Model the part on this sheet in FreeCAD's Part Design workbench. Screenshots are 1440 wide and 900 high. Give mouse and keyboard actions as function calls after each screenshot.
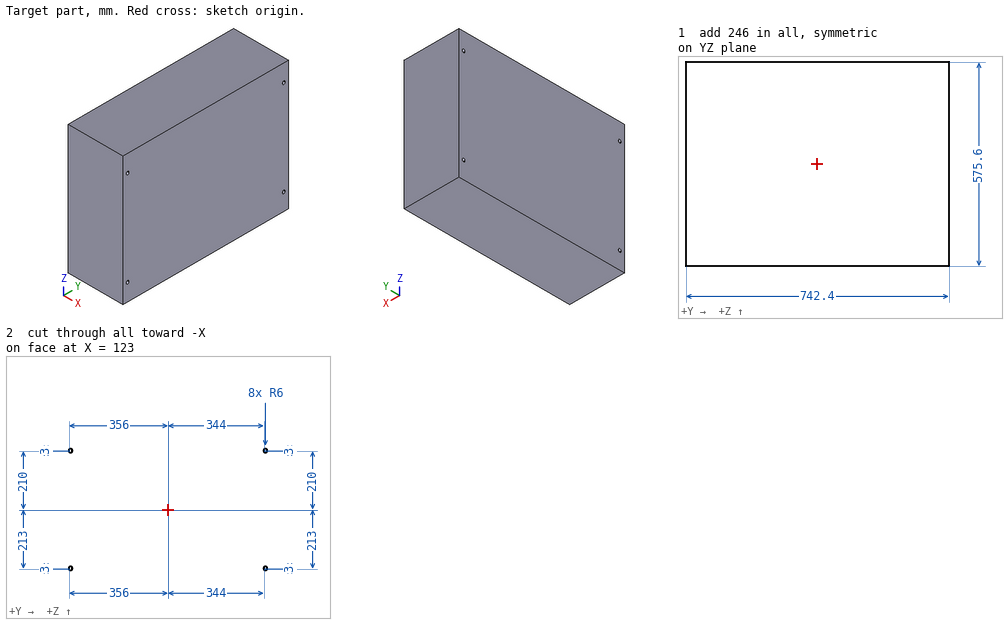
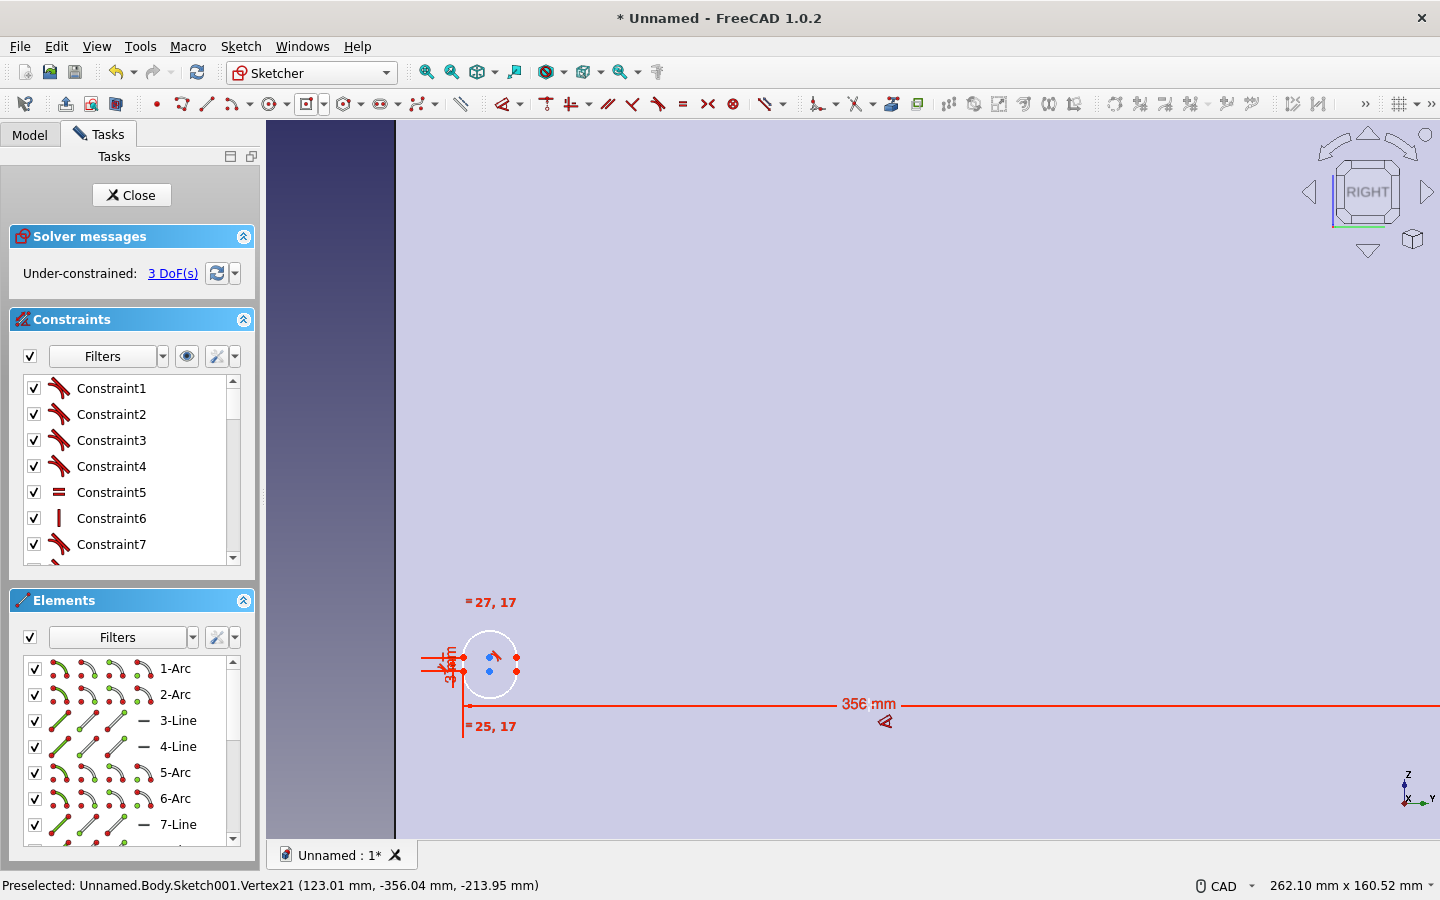
click(463, 671)
click(429, 410)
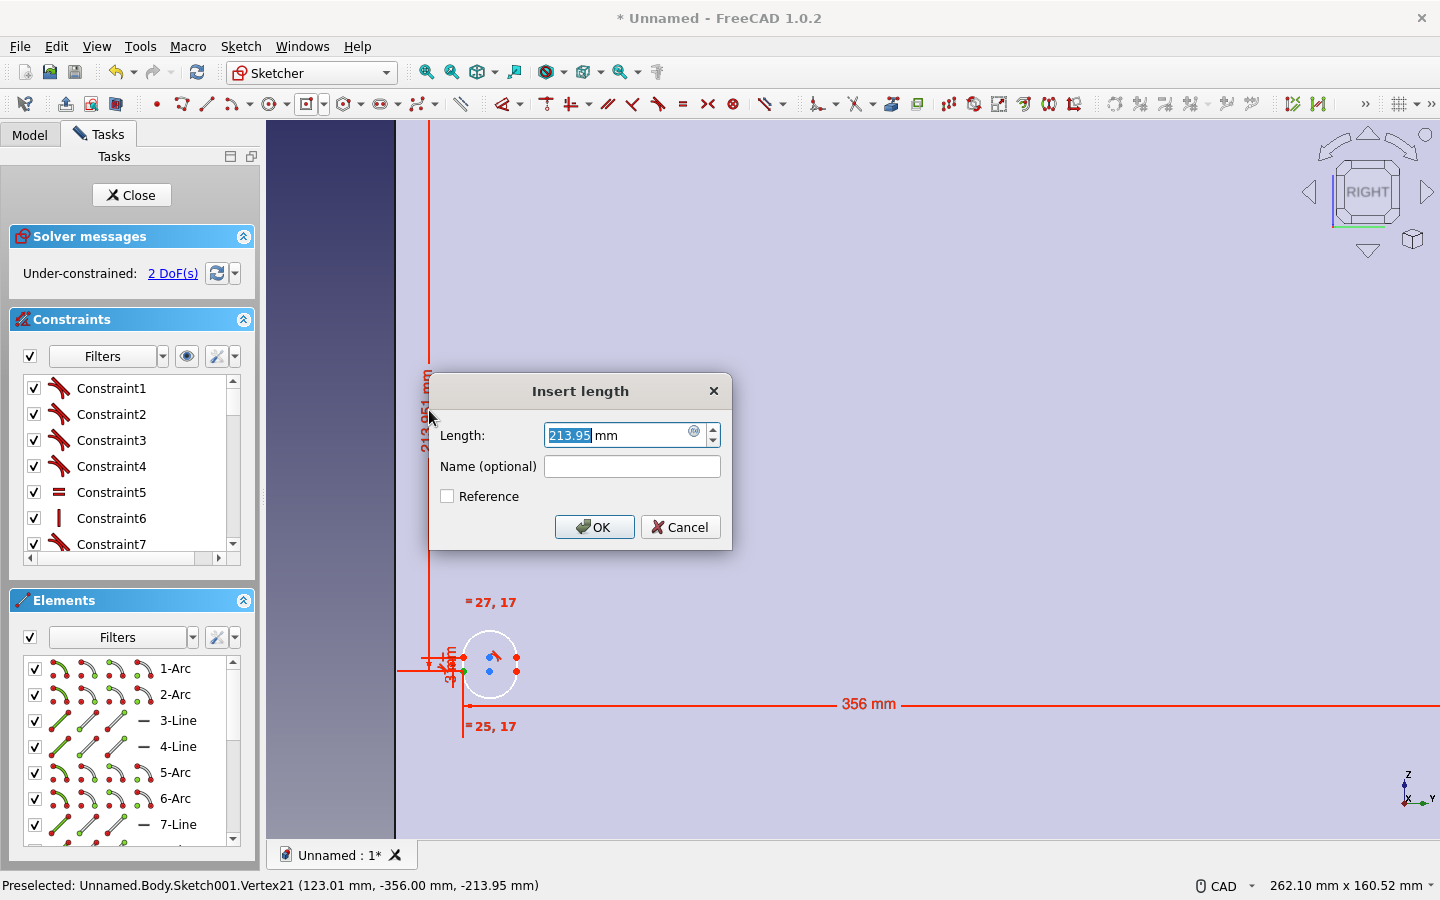
text(213)
key(Return)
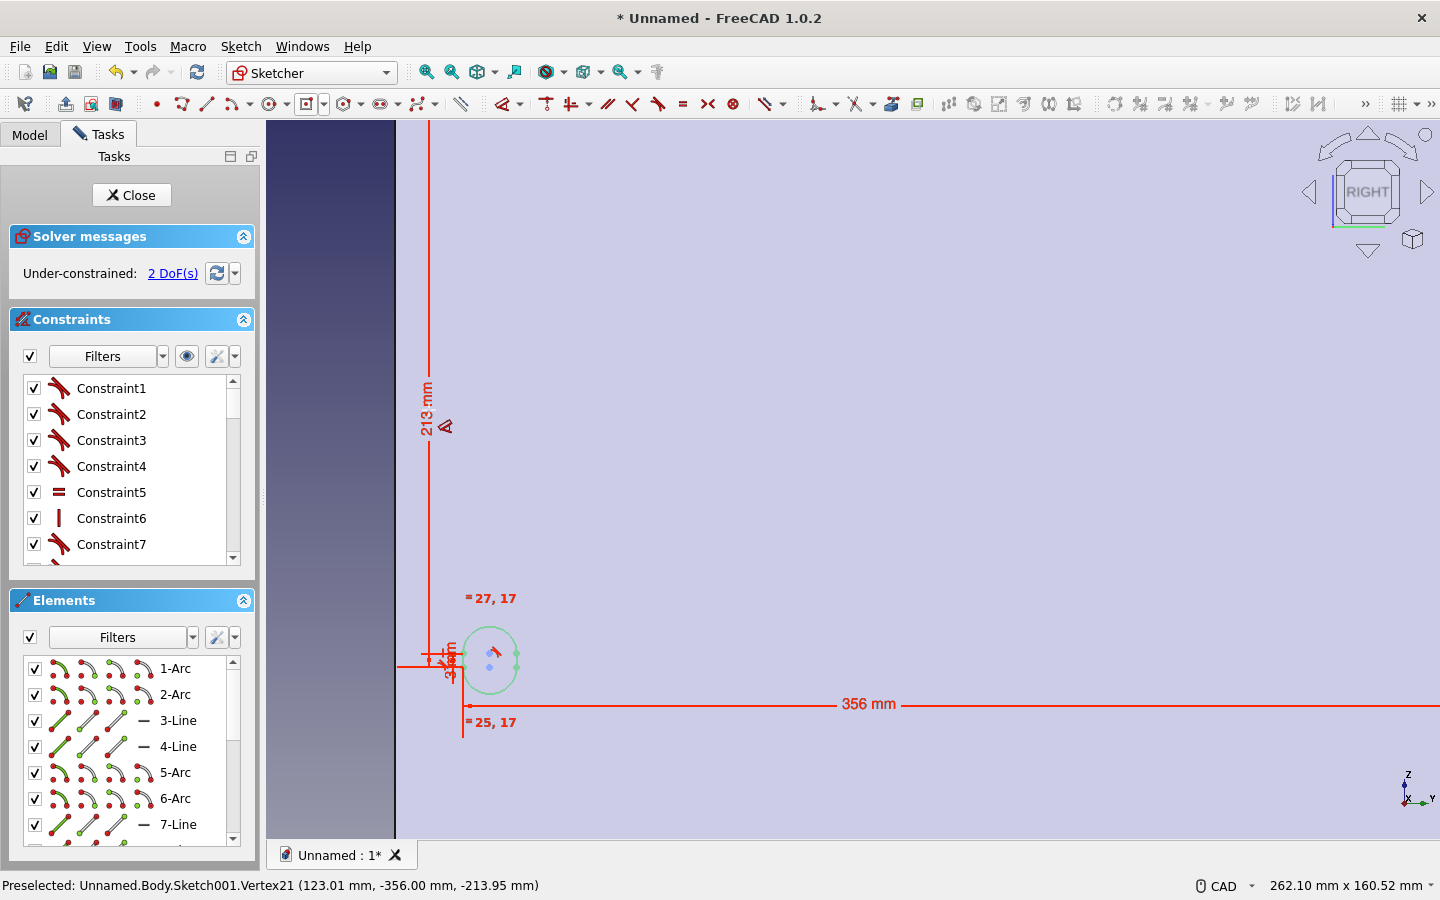
scroll(462, 673, down, 8)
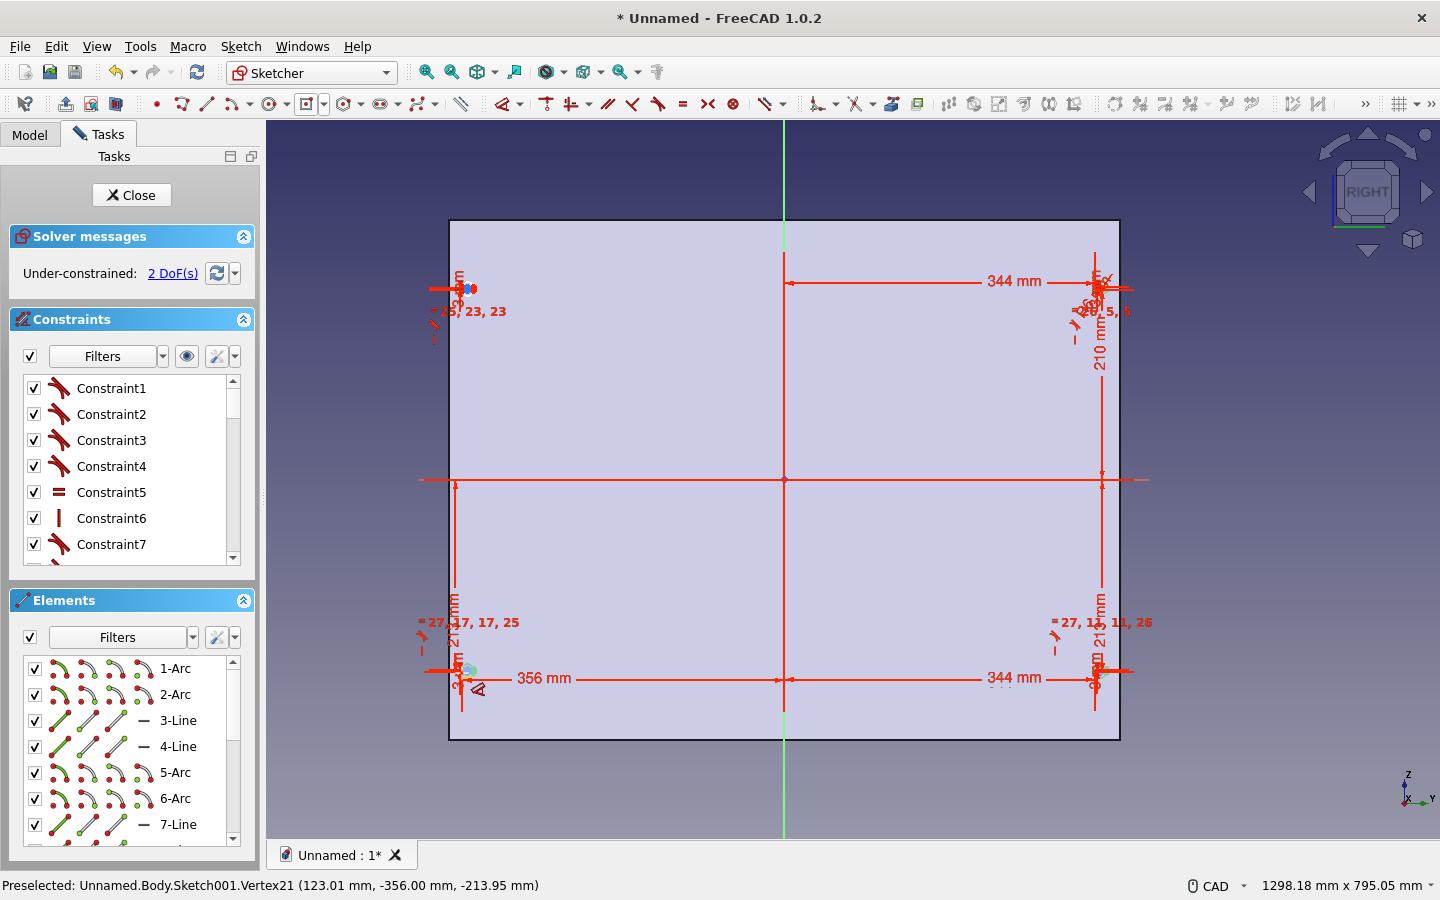
scroll(463, 290, up, 8)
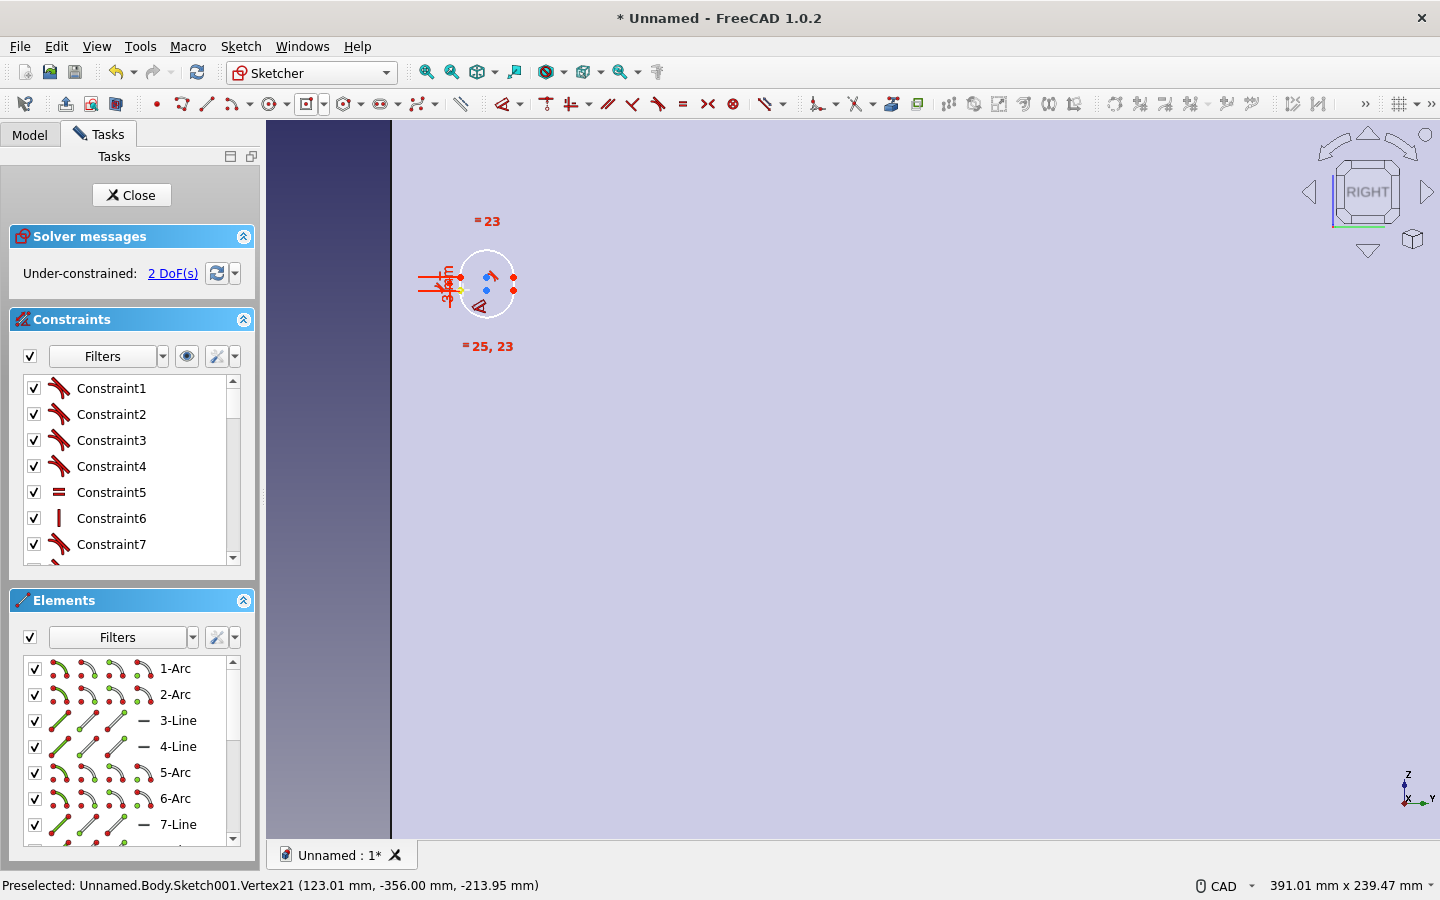
click(460, 291)
click(868, 257)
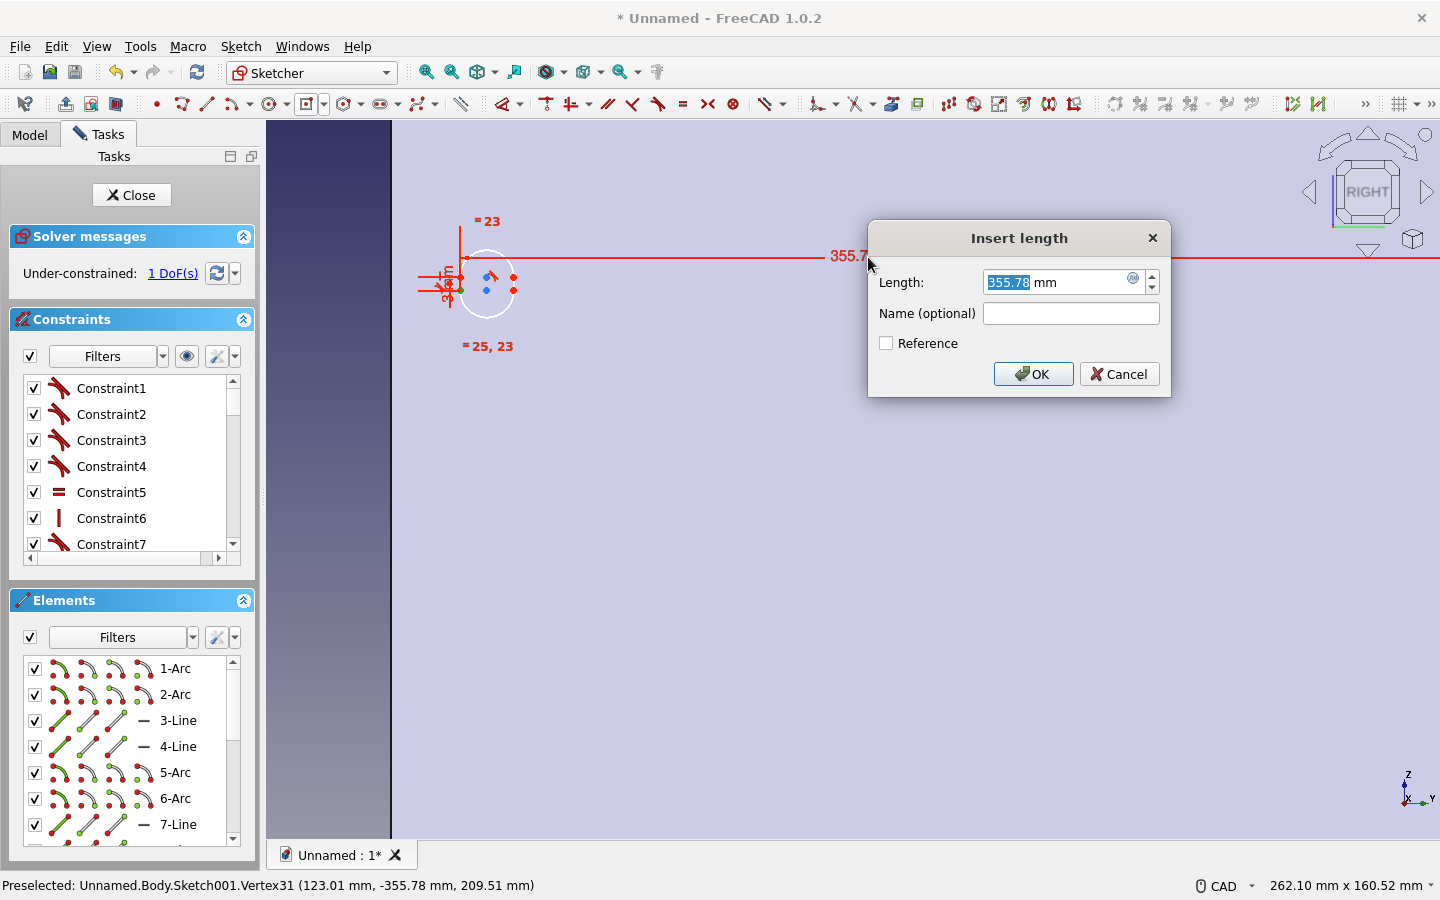
text(356)
key(Return)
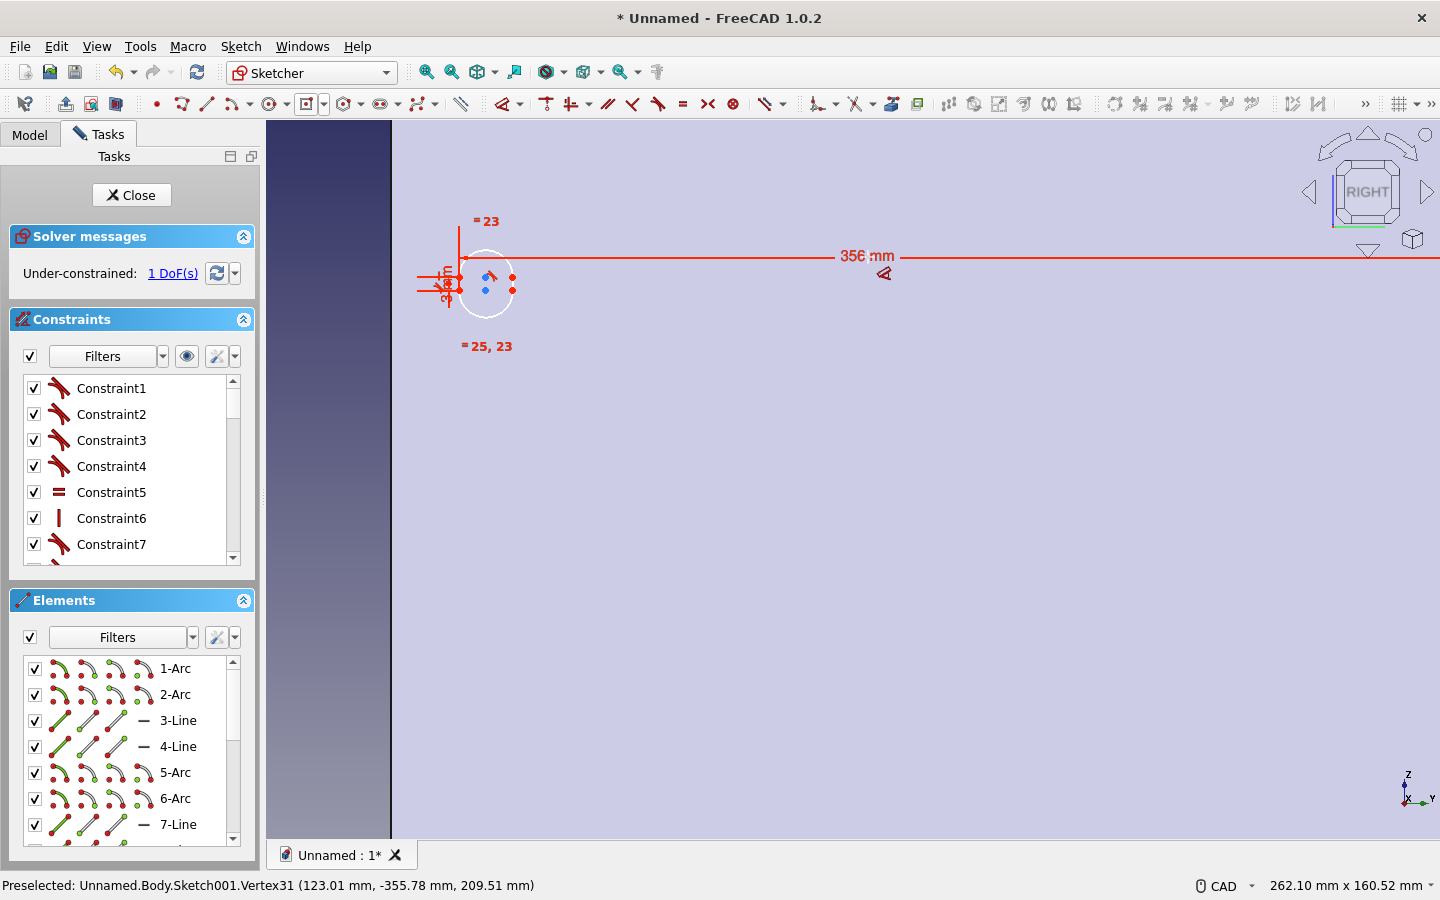
click(459, 291)
click(425, 551)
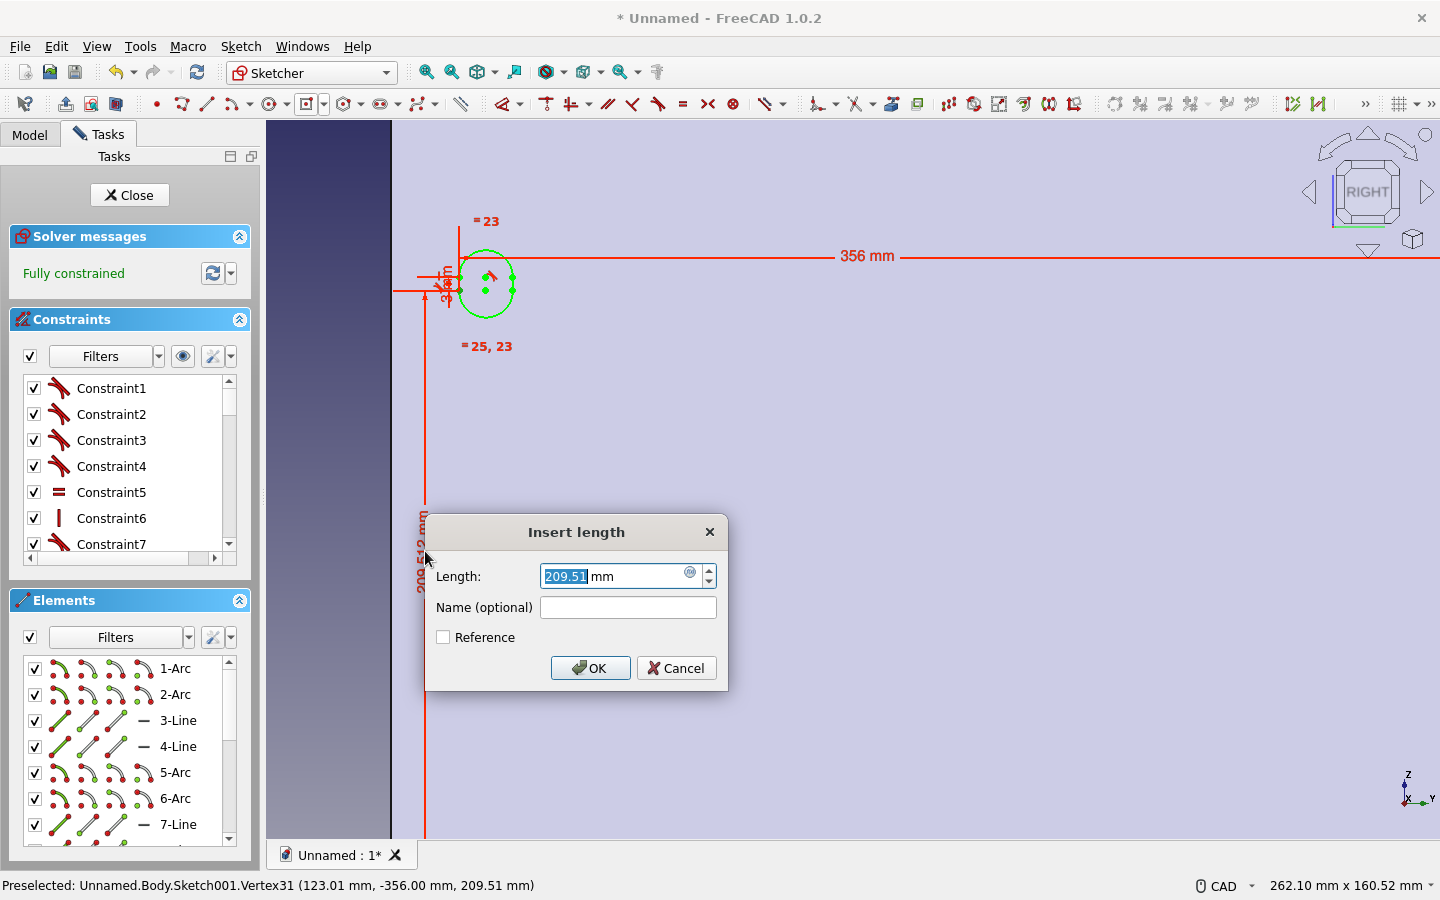
text(210)
key(Return)
key(Escape)